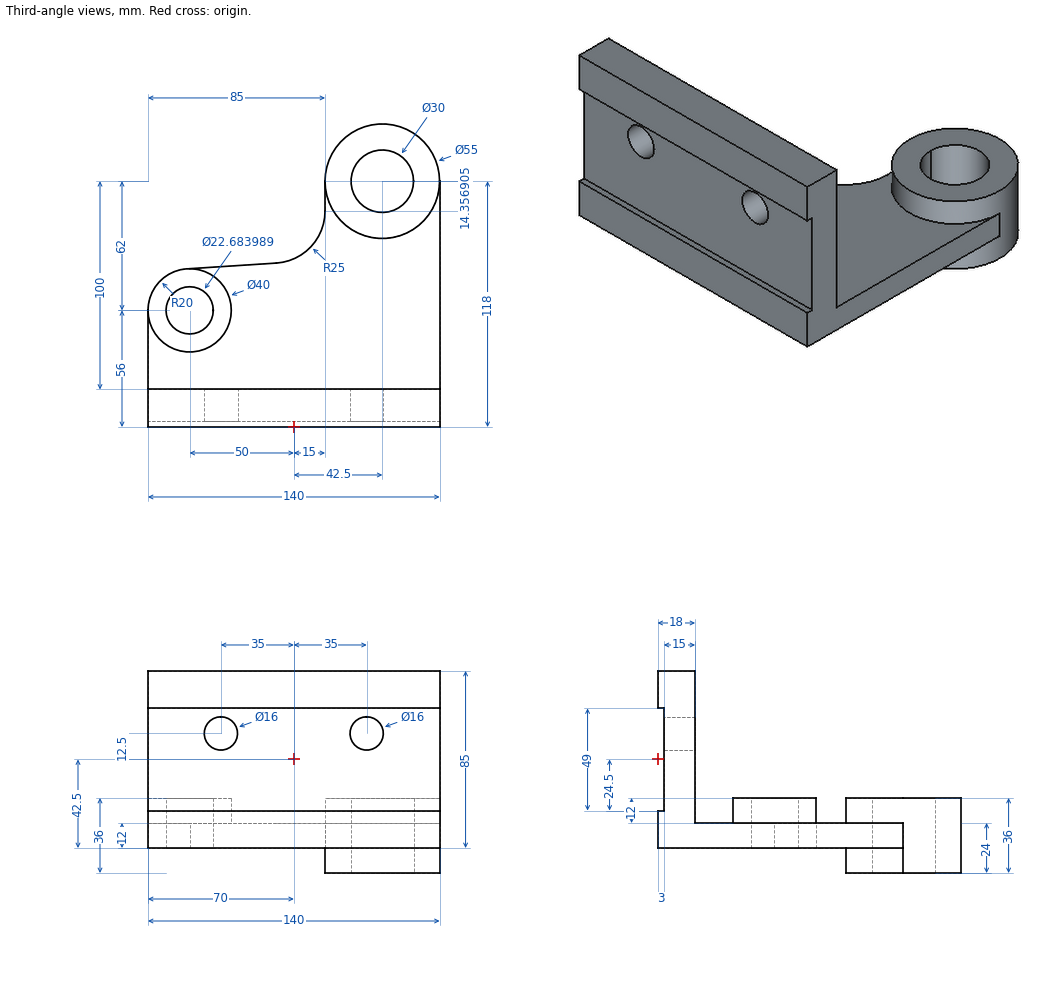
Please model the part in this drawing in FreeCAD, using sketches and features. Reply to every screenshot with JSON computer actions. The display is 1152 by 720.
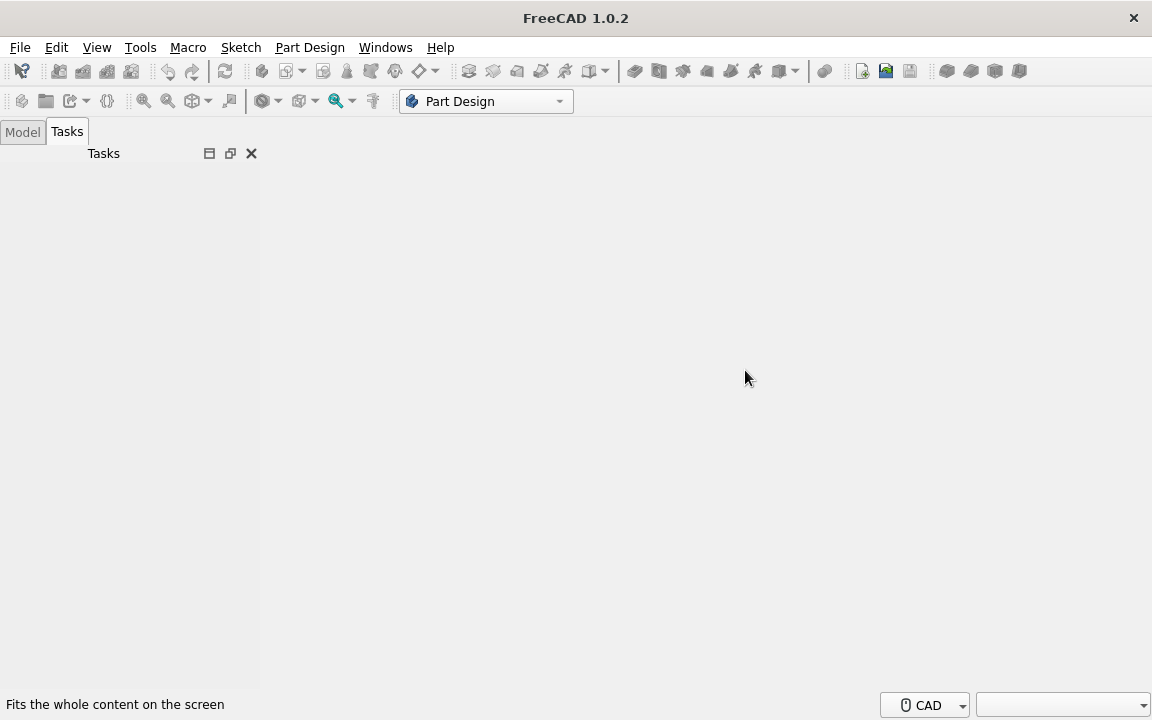
{"action": "left_click", "coordinate": [862, 72]}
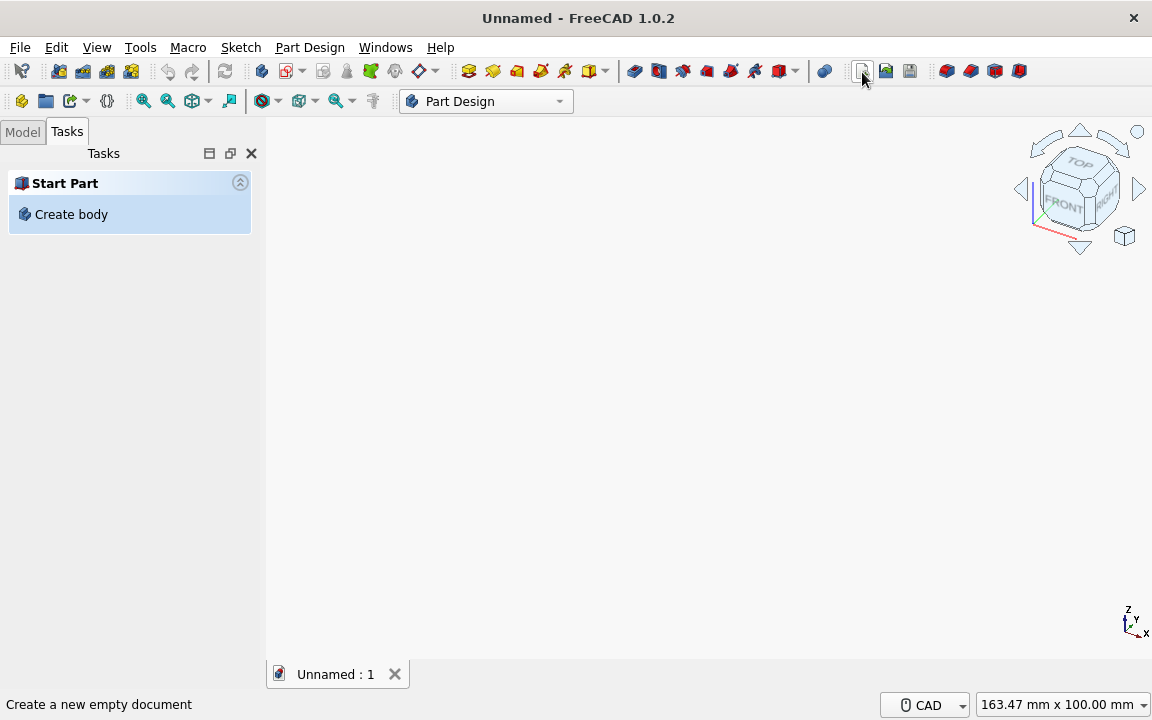
{"action": "left_click", "coordinate": [286, 72]}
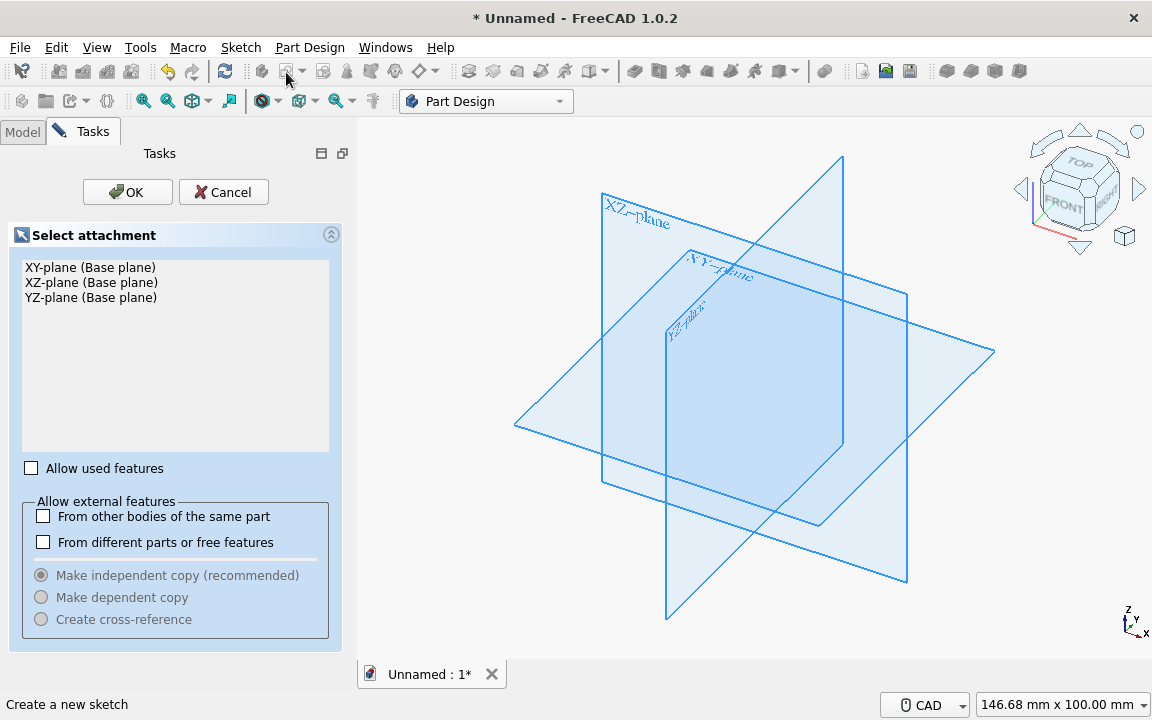
{"action": "left_click", "coordinate": [82, 282]}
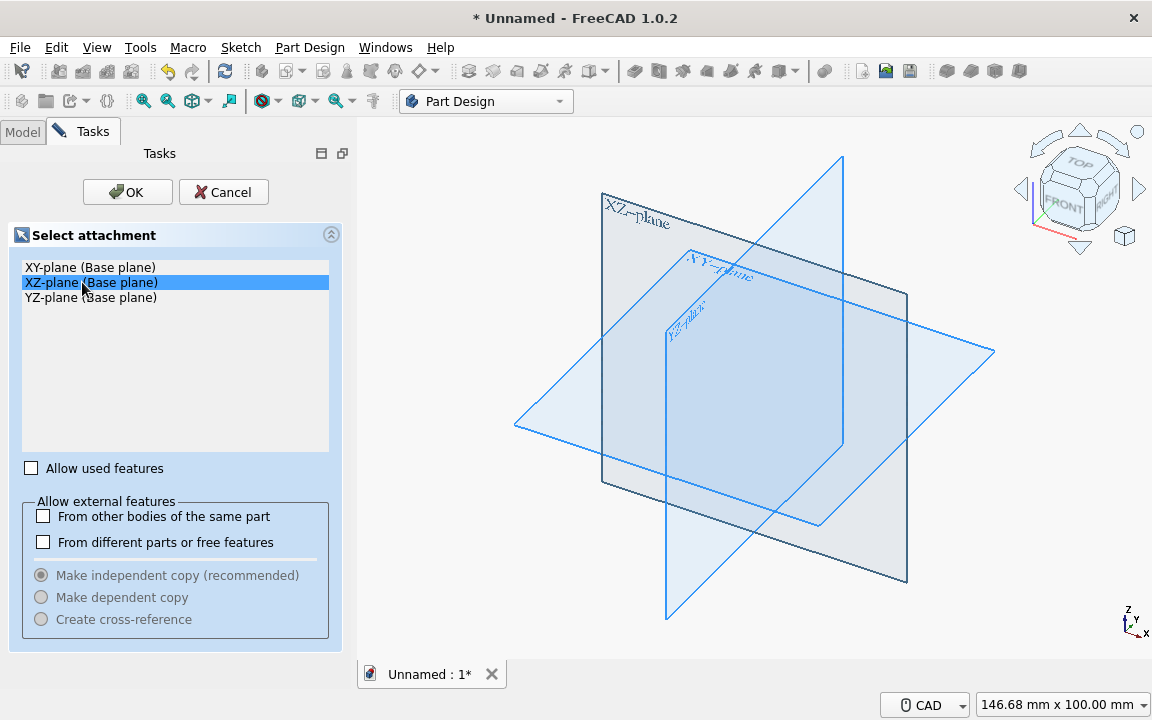
{"action": "left_click", "coordinate": [128, 192]}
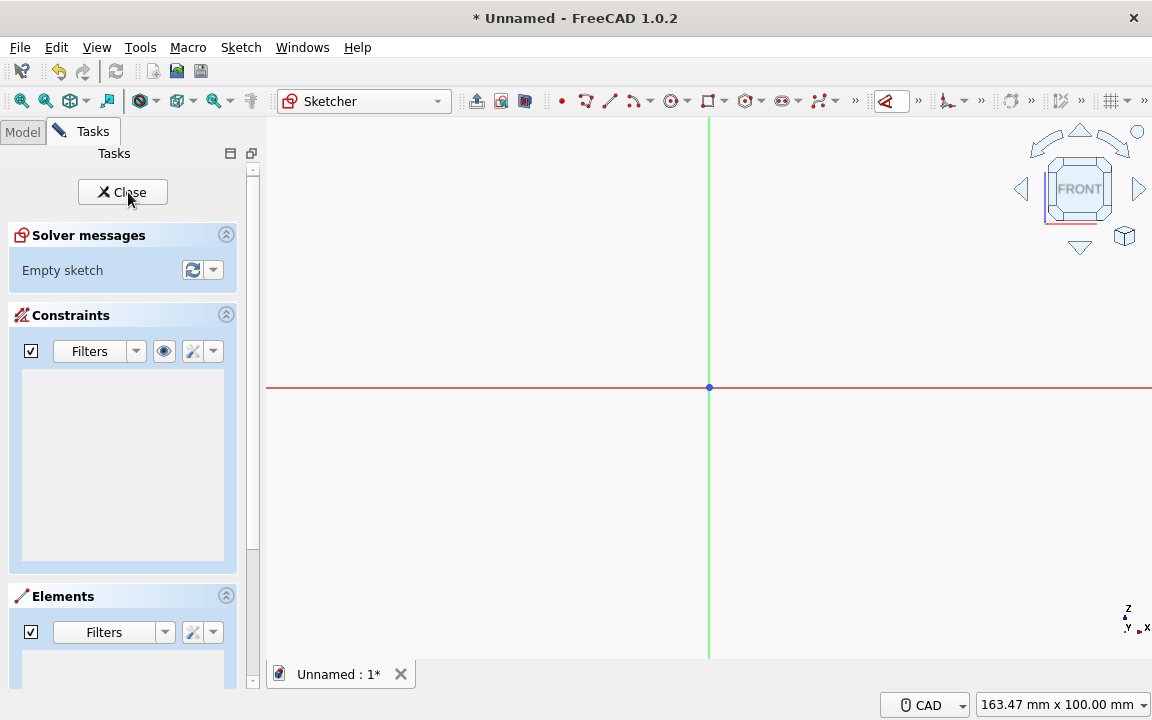
{"action": "scroll", "coordinate": [501, 388], "scroll_direction": "down", "scroll_amount": 2}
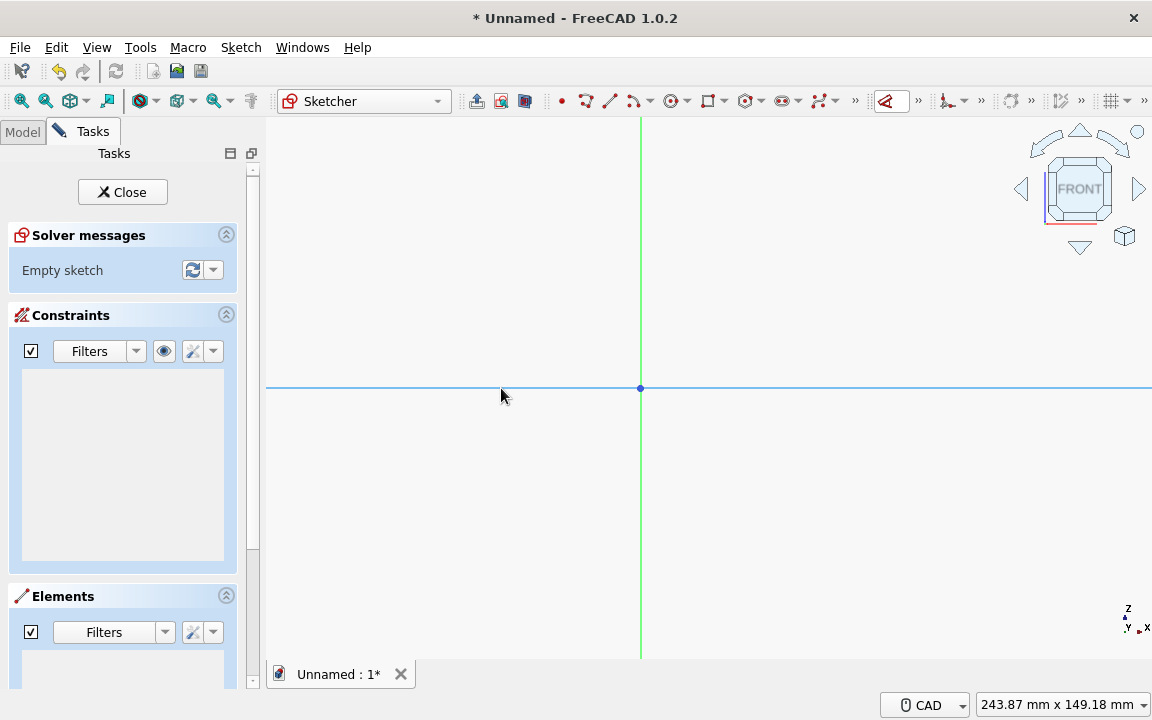
{"action": "left_click", "coordinate": [726, 102]}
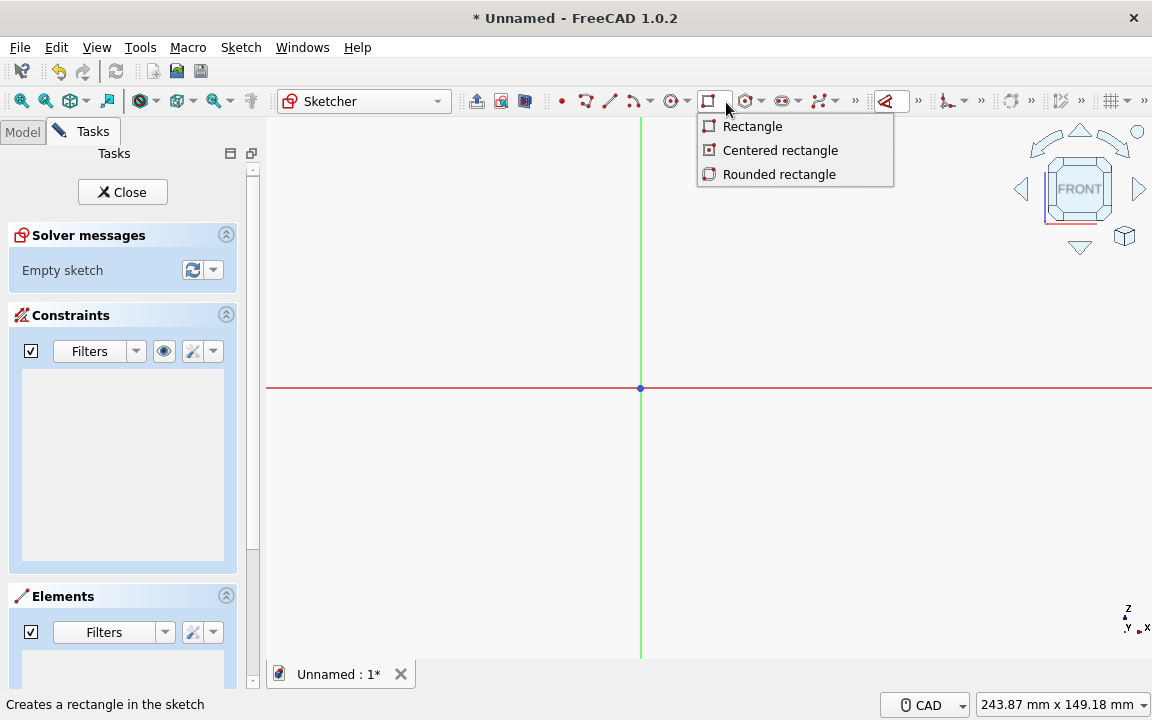
{"action": "left_click", "coordinate": [796, 150]}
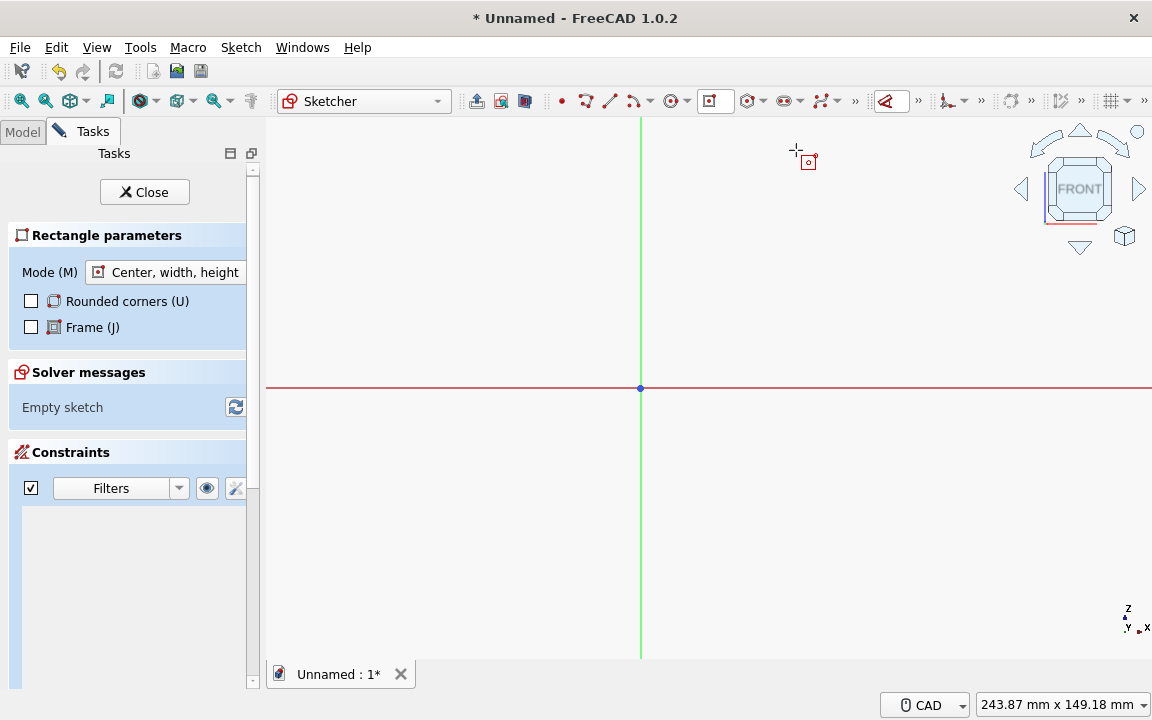
{"action": "left_click", "coordinate": [641, 388]}
{"action": "left_click", "coordinate": [895, 234]}
{"action": "key", "text": "Escape"}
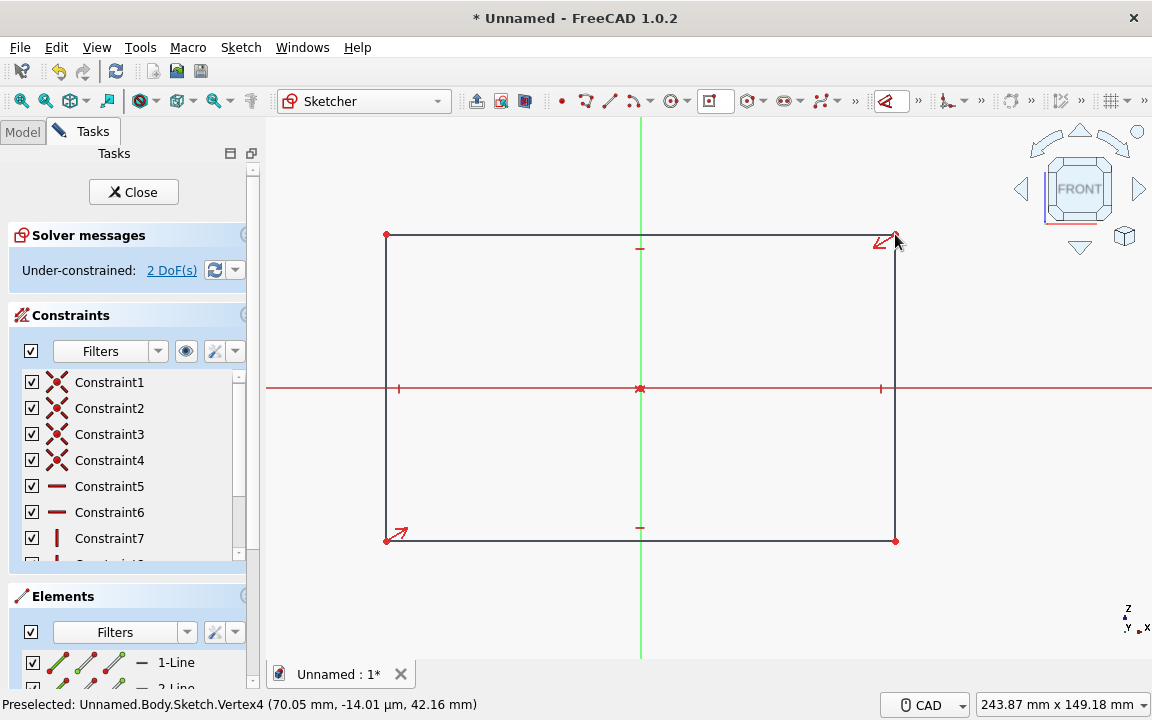
{"action": "left_click", "coordinate": [895, 449]}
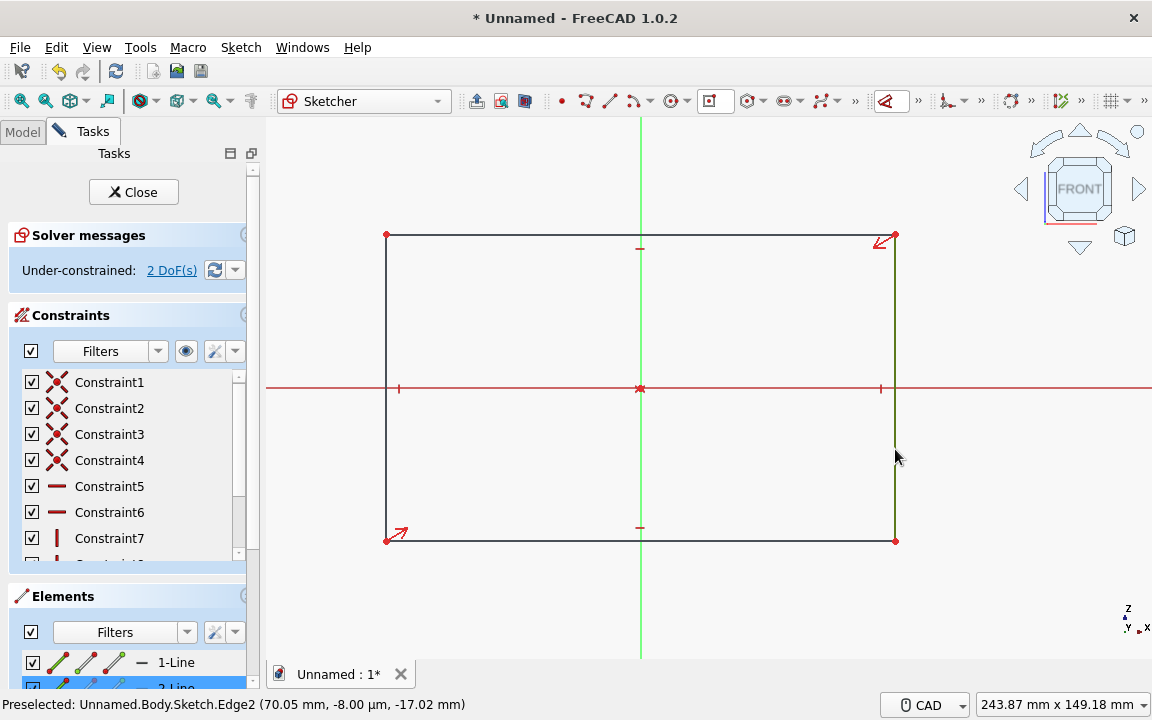
{"action": "key", "text": "i"}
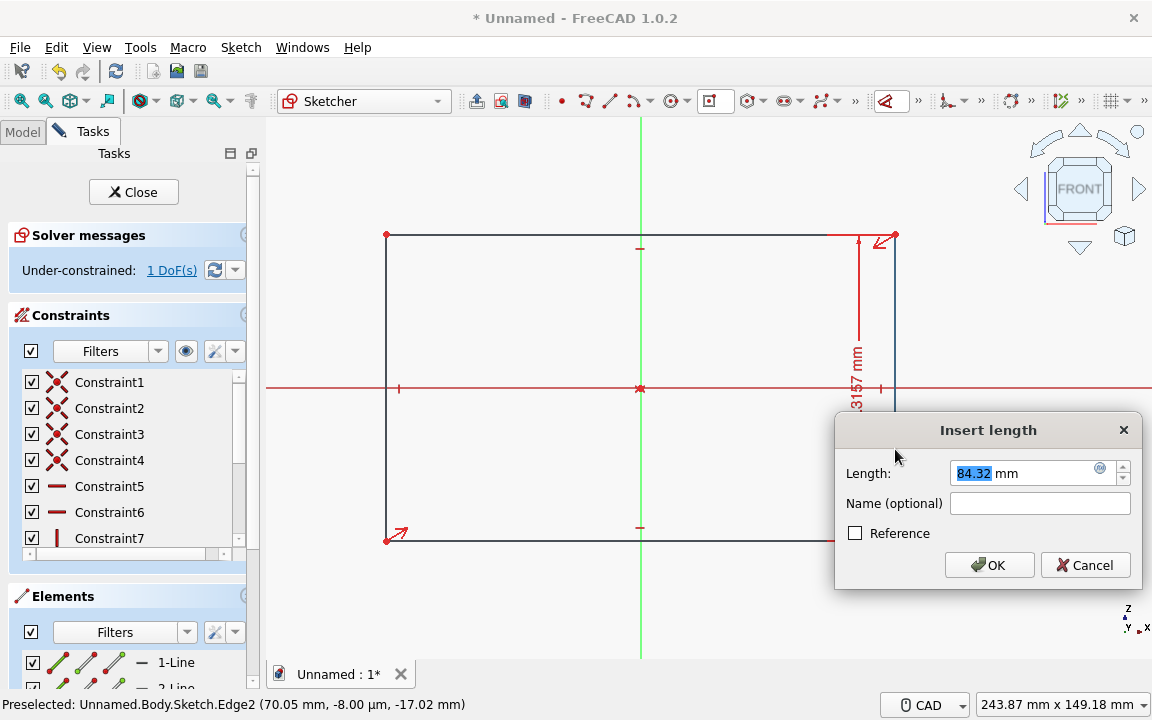
{"action": "type", "text": "85"}
{"action": "key", "text": "Return"}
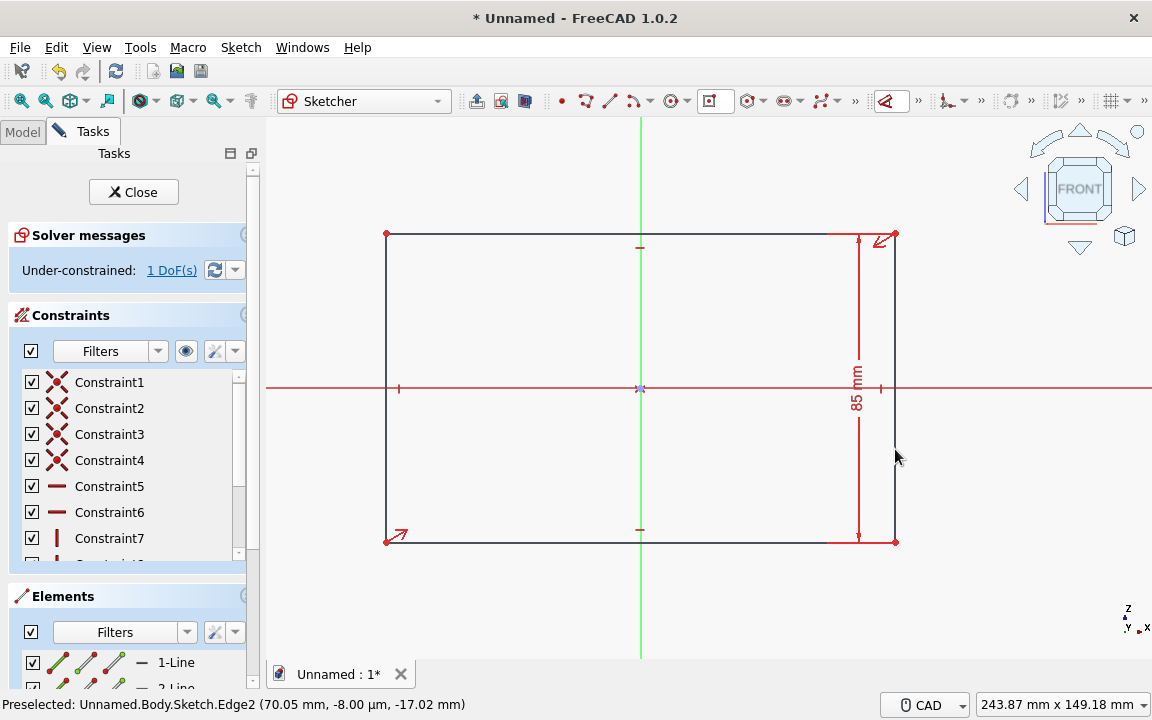
{"action": "left_click", "coordinate": [539, 543]}